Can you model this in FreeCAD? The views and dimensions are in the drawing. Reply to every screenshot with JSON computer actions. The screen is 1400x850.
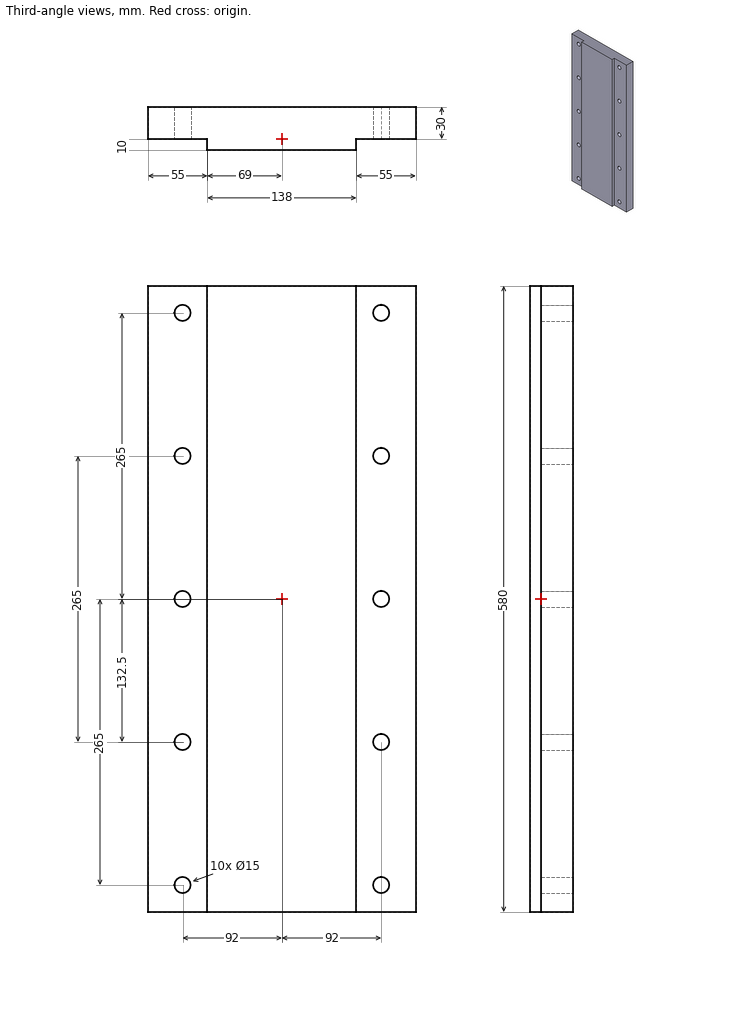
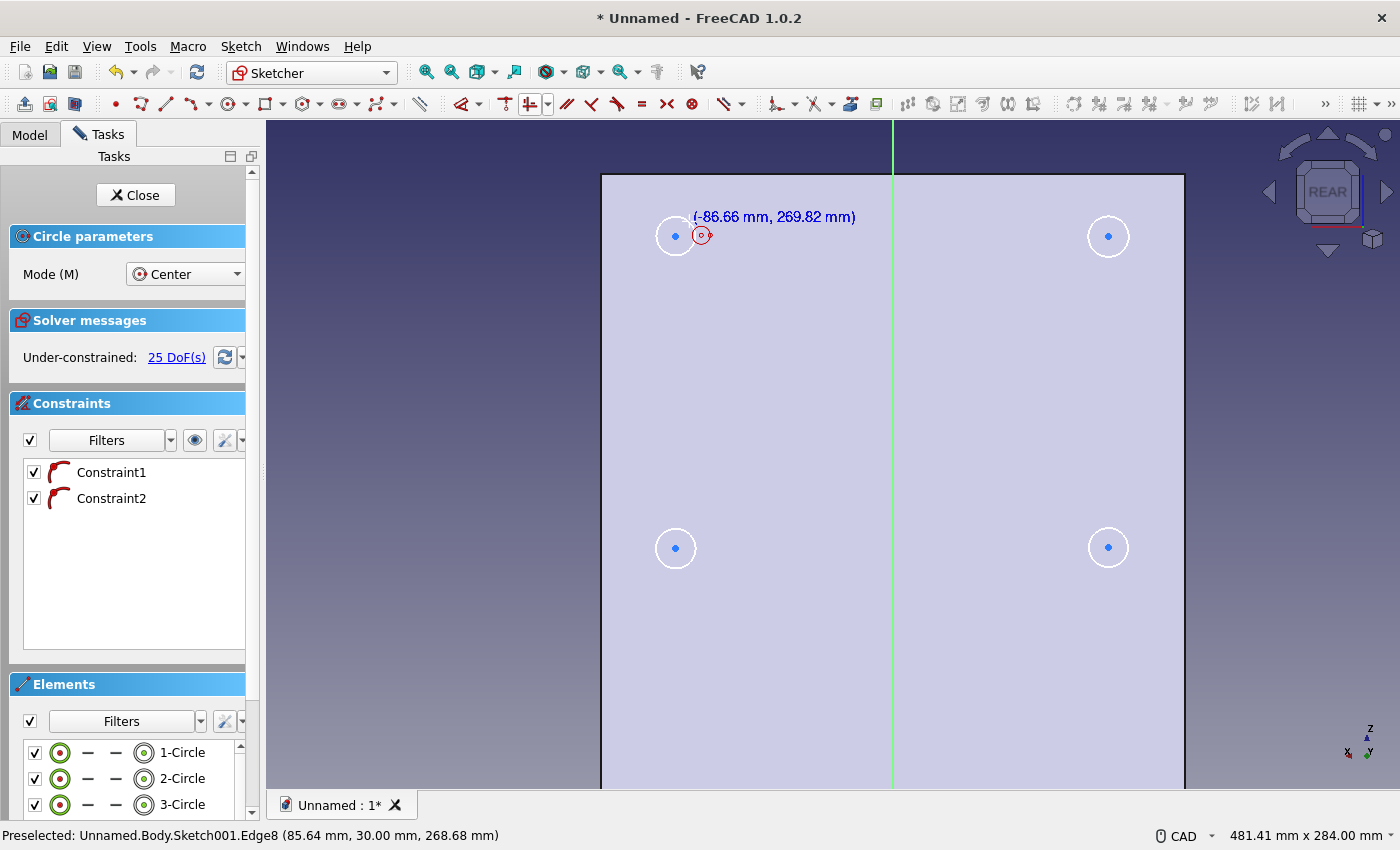
{"action": "scroll", "coordinate": [690, 220], "scroll_direction": "down", "scroll_amount": 5}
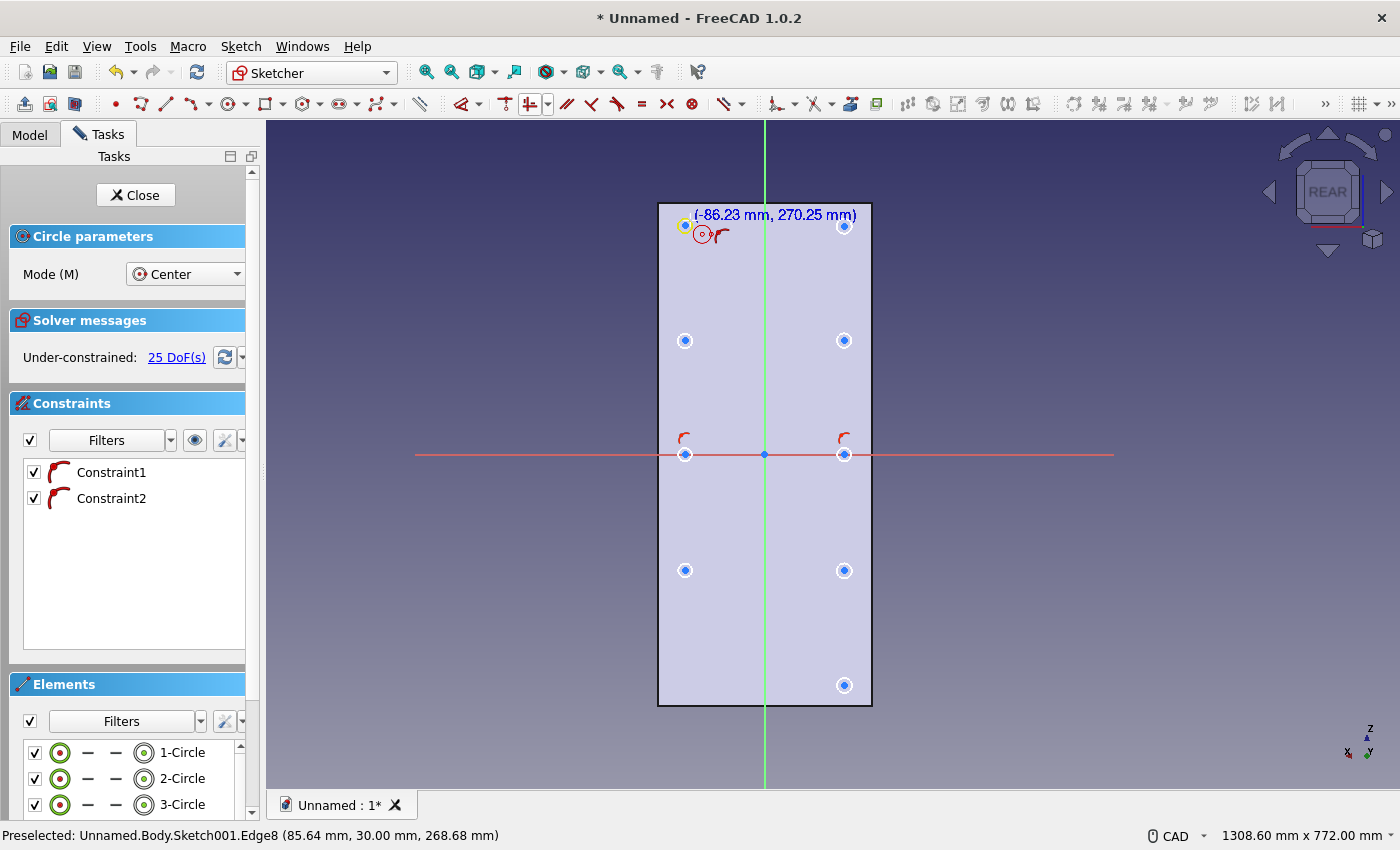
{"action": "scroll", "coordinate": [685, 684], "scroll_direction": "up", "scroll_amount": 7}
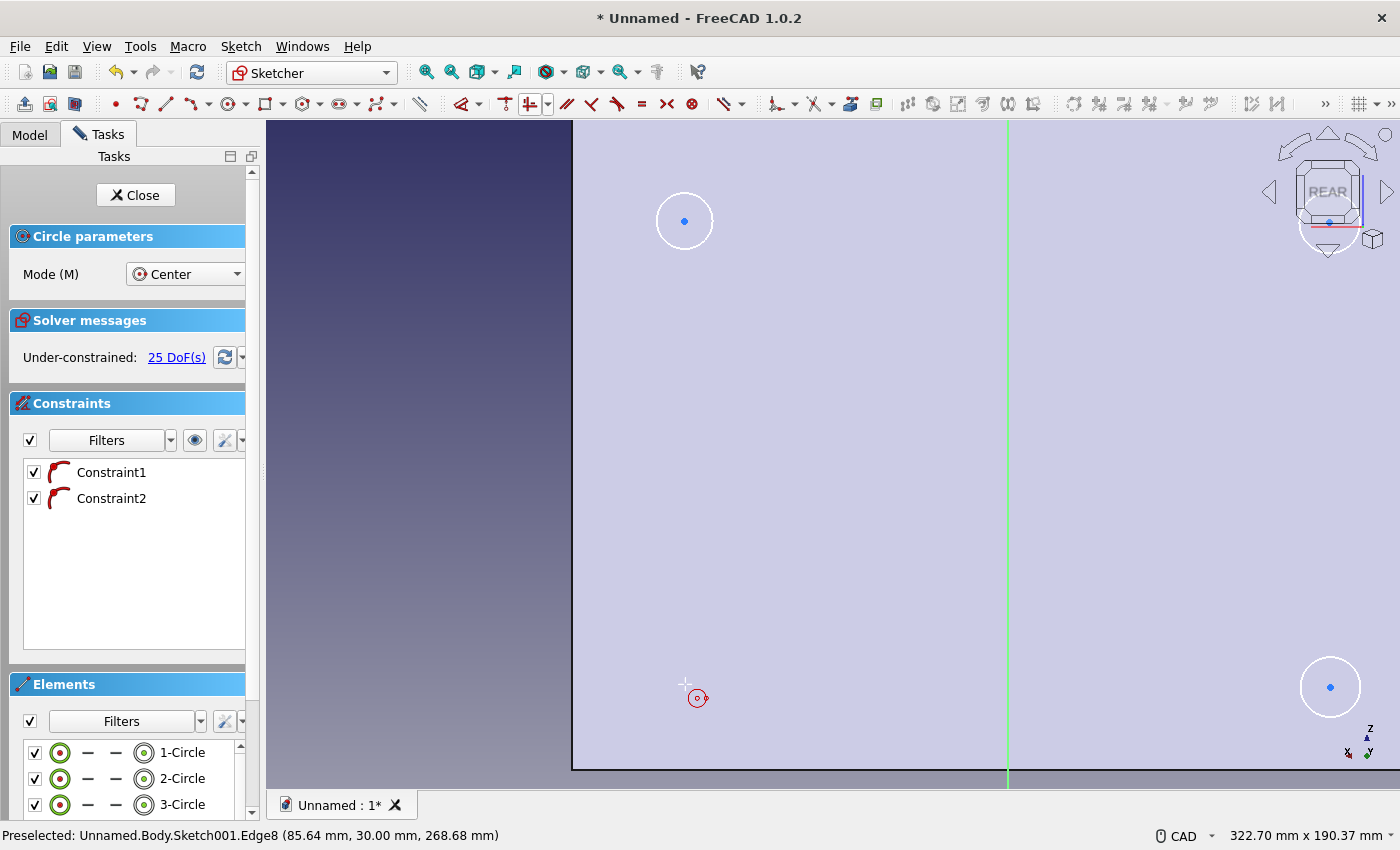
{"action": "scroll", "coordinate": [685, 685], "scroll_direction": "down", "scroll_amount": 7}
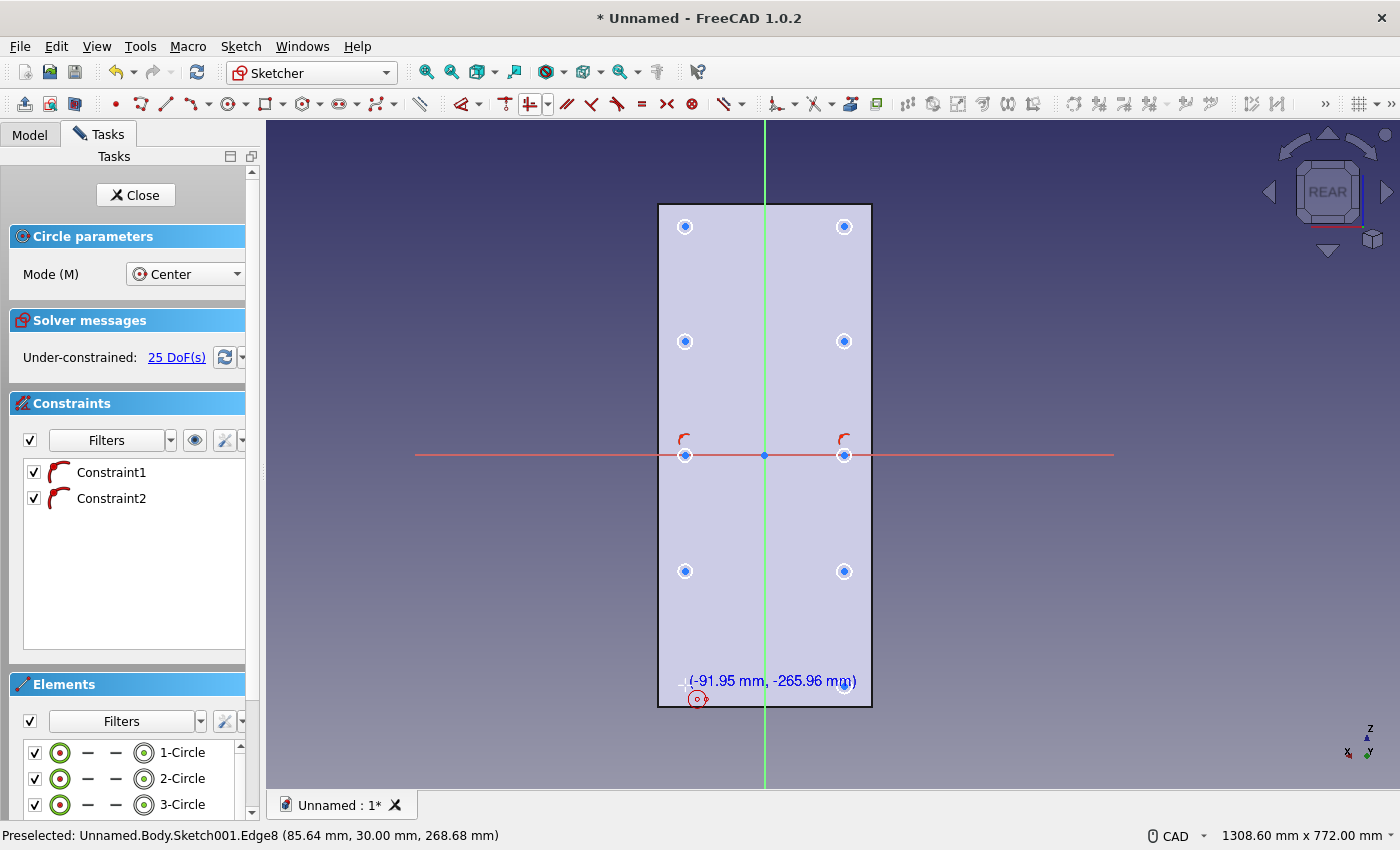
{"action": "left_click", "coordinate": [685, 685]}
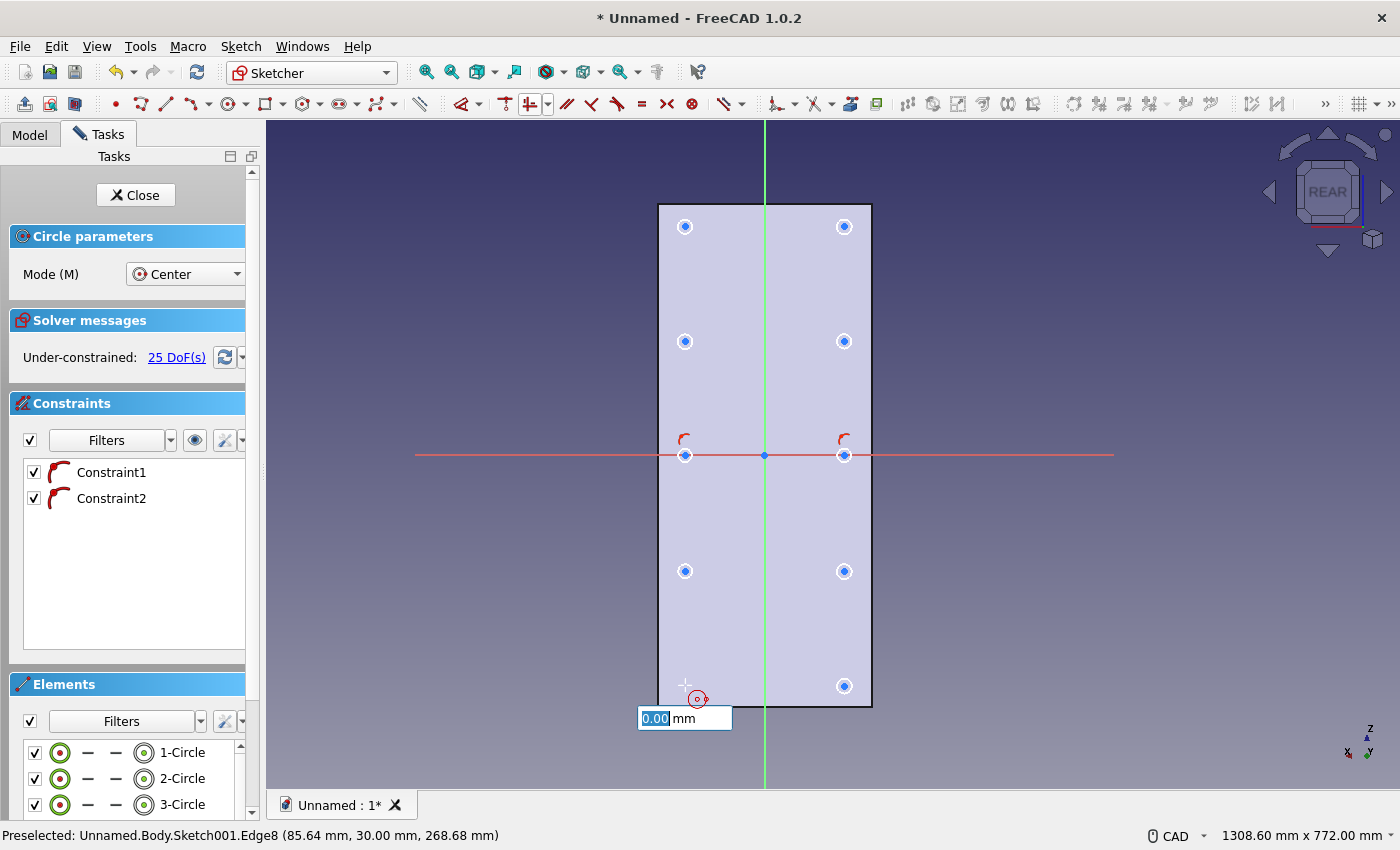
{"action": "scroll", "coordinate": [690, 680], "scroll_direction": "up", "scroll_amount": 5}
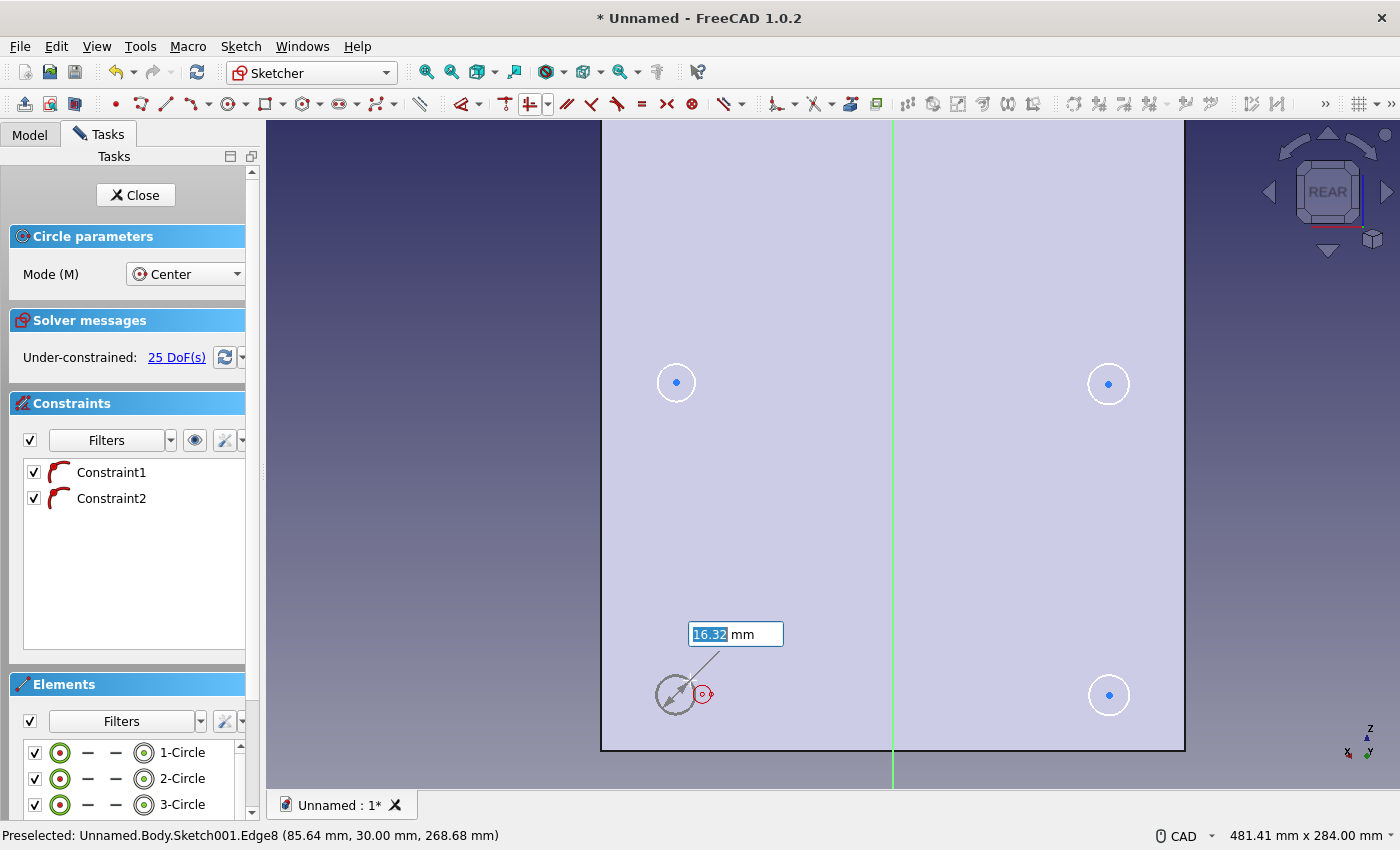
{"action": "left_click", "coordinate": [689, 680]}
{"action": "key", "text": "Escape"}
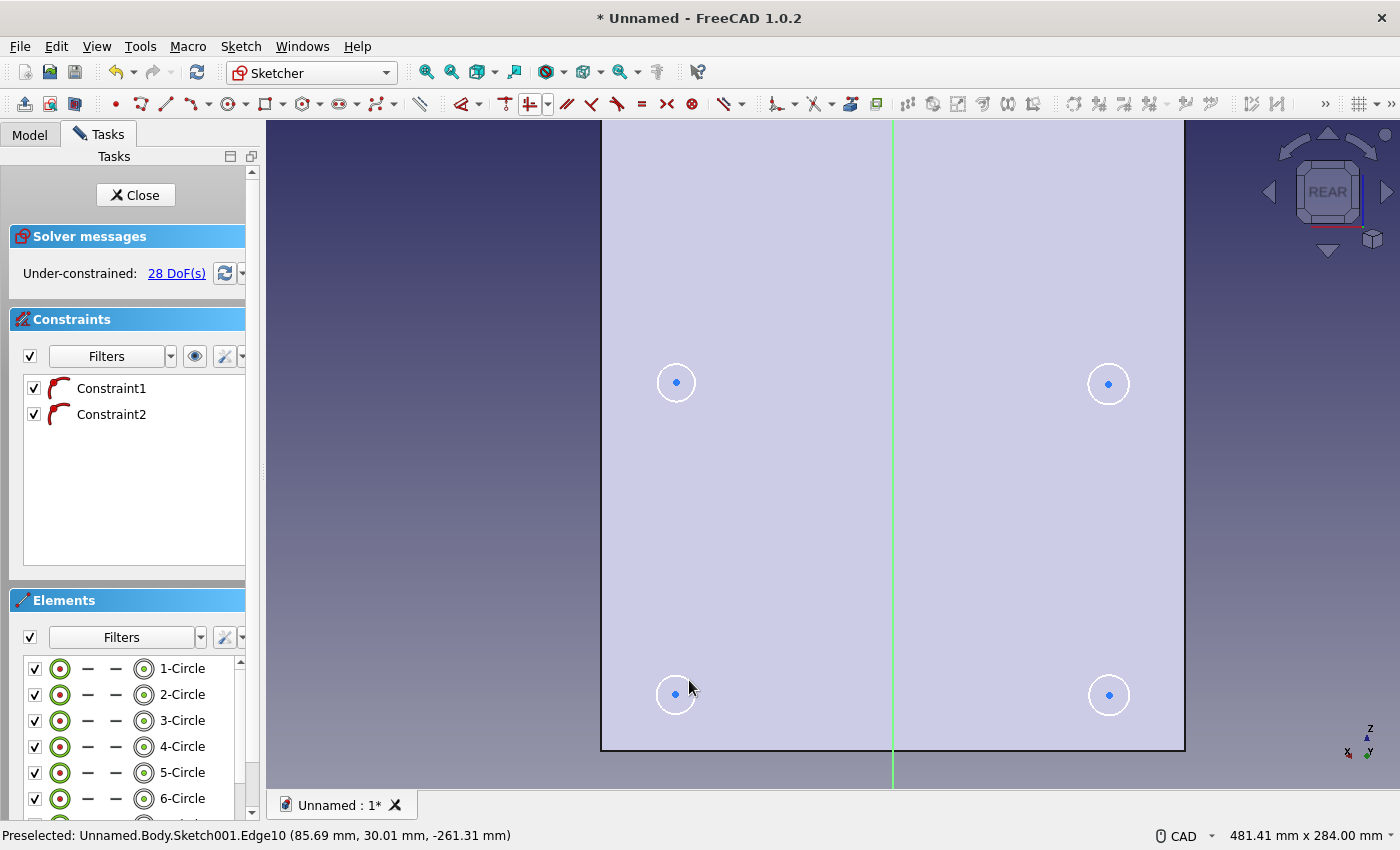
{"action": "left_click", "coordinate": [1123, 681]}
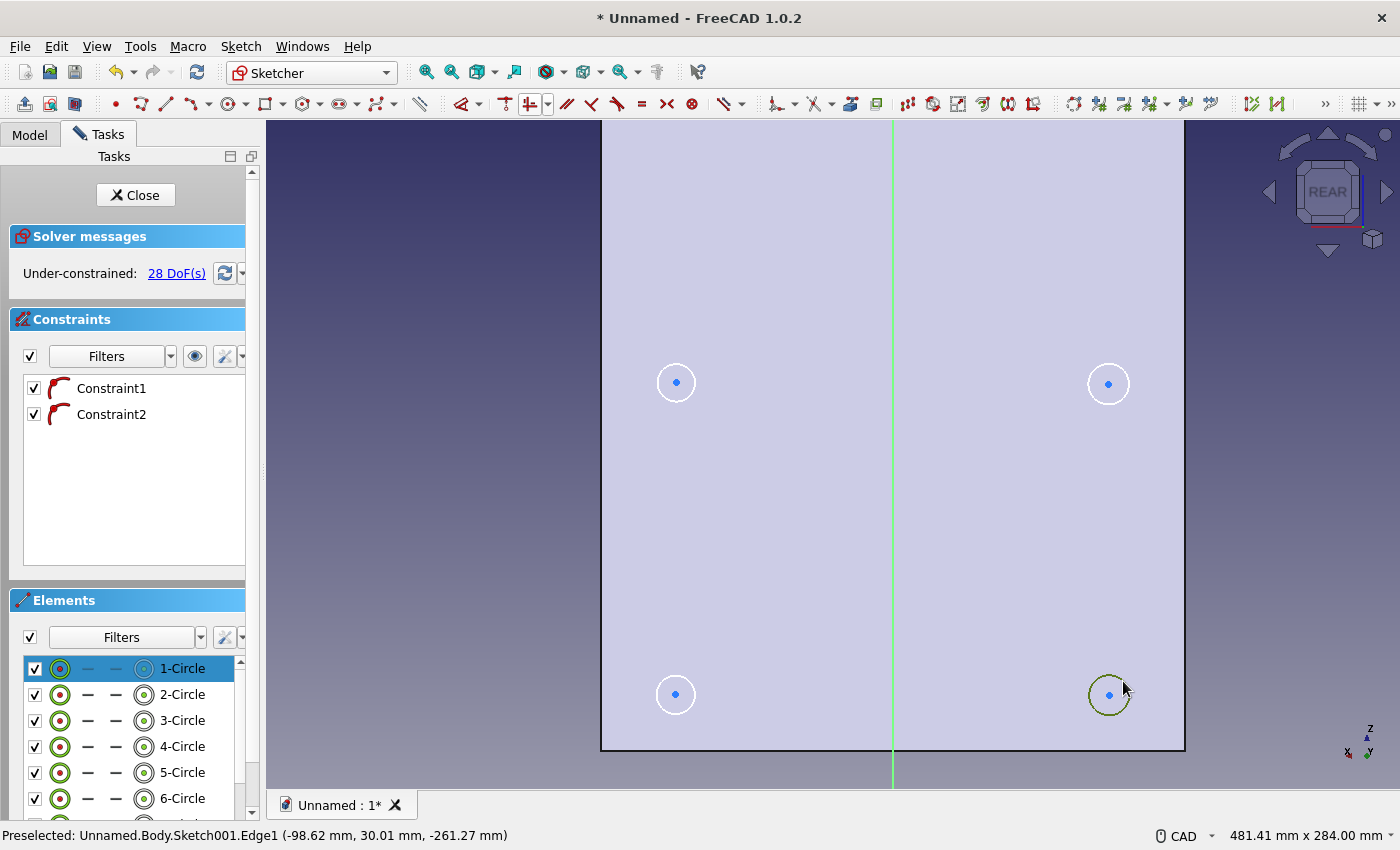
{"action": "left_click", "coordinate": [1123, 370]}